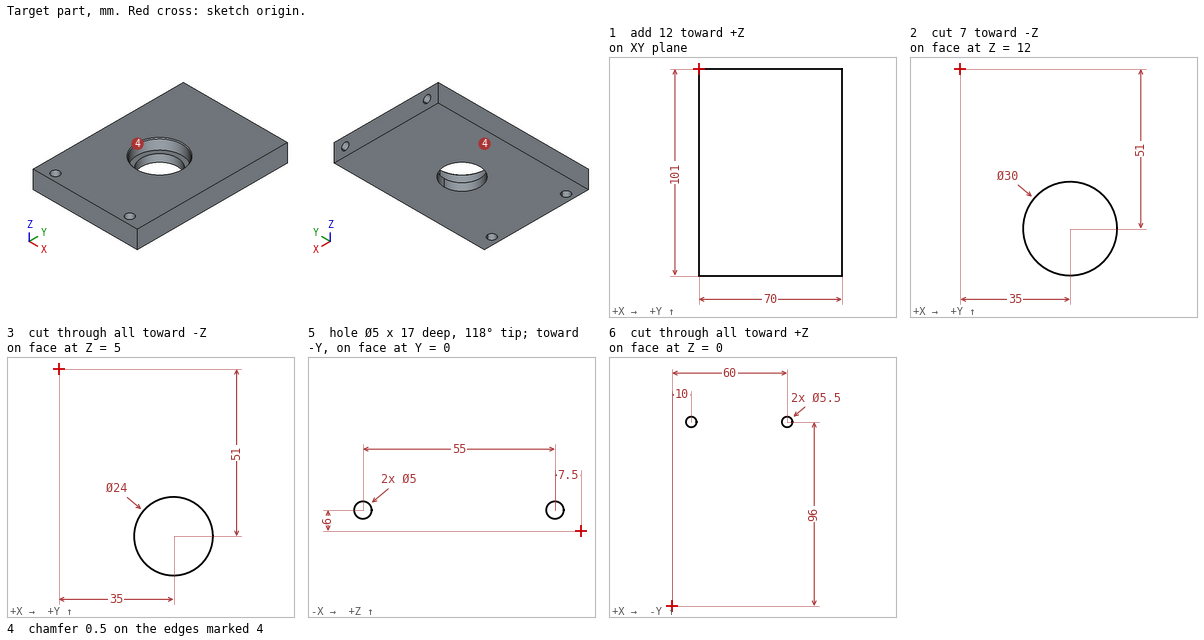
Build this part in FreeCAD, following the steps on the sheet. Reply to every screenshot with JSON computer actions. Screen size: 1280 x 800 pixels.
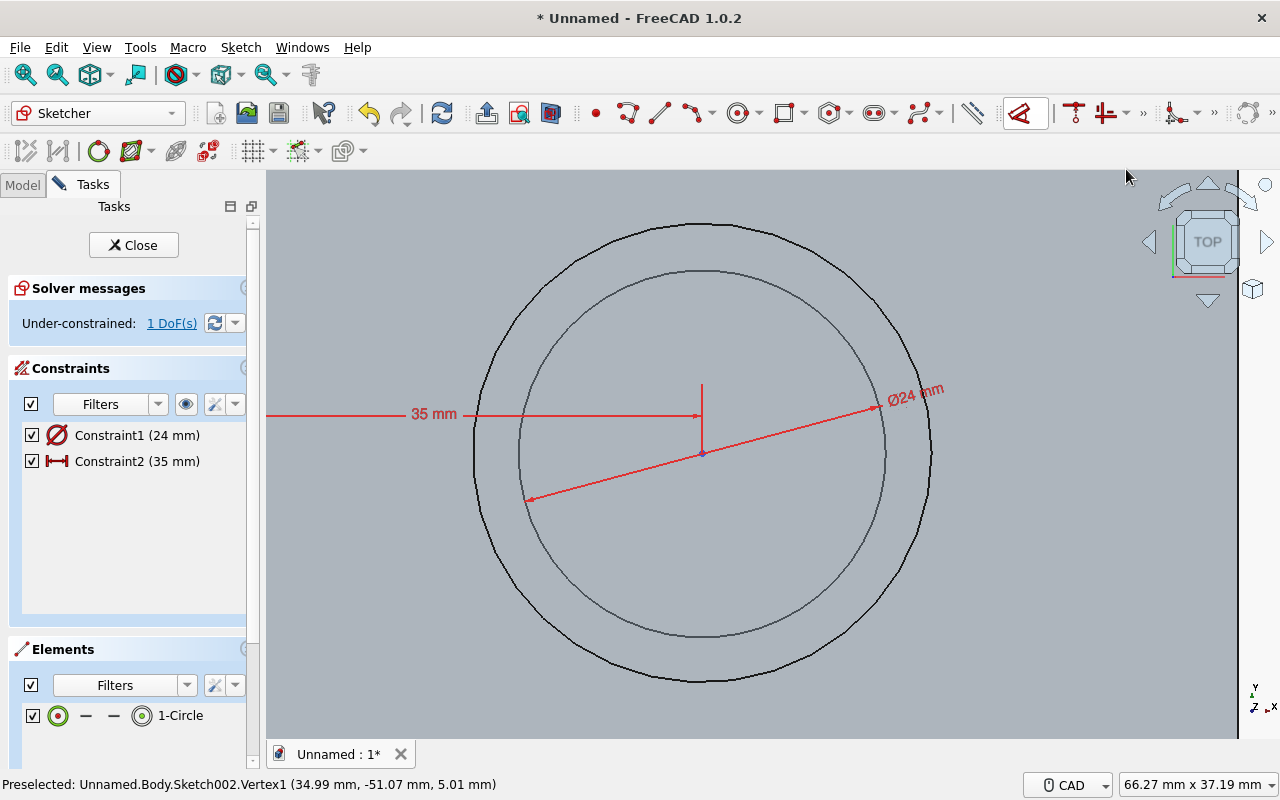
{"action": "left_click", "coordinate": [702, 454]}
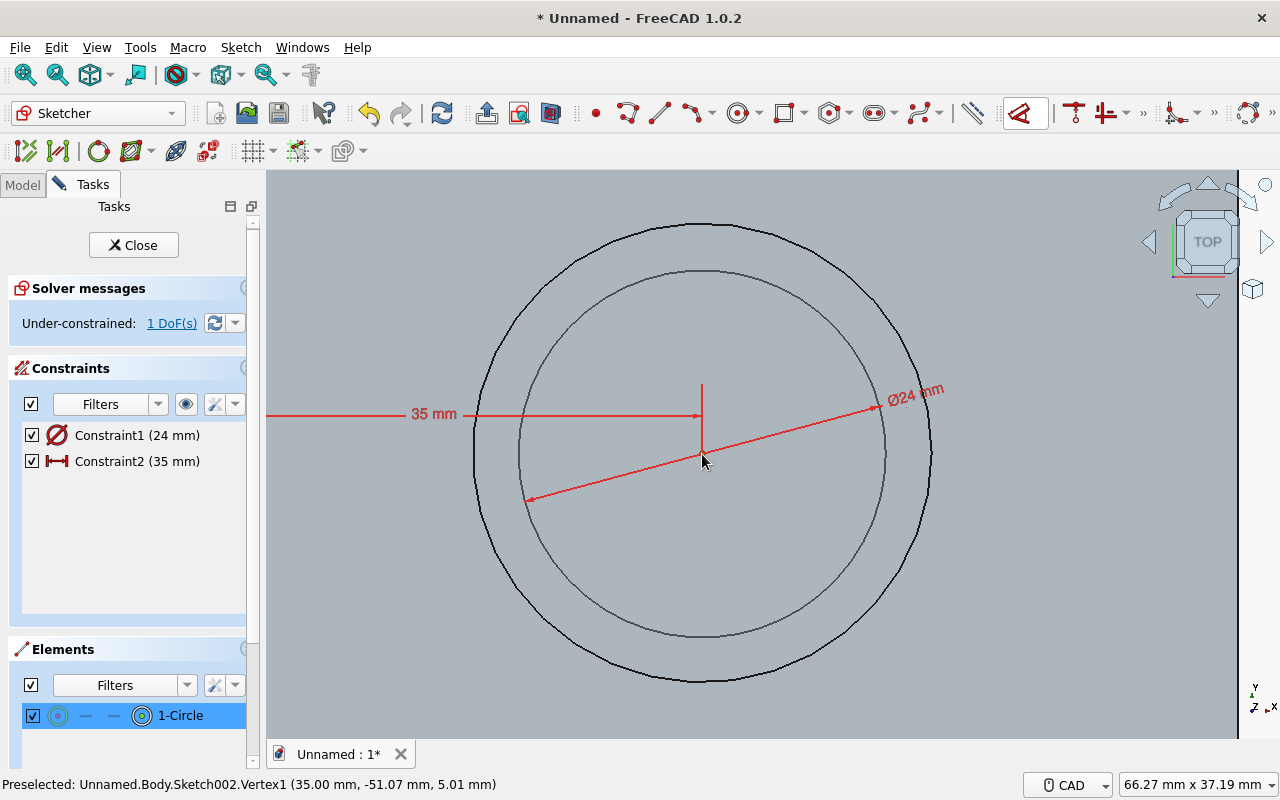
{"action": "left_click", "coordinate": [1042, 114]}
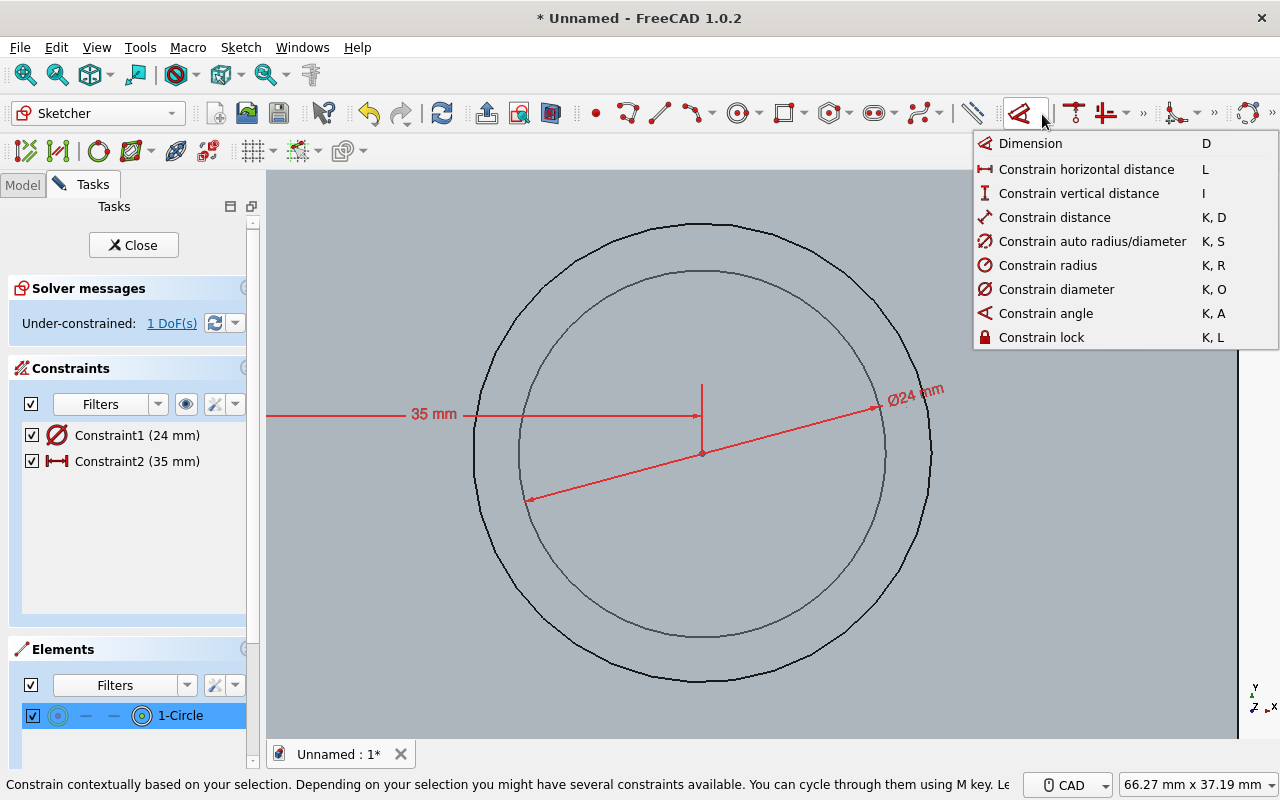
{"action": "left_click", "coordinate": [1126, 193]}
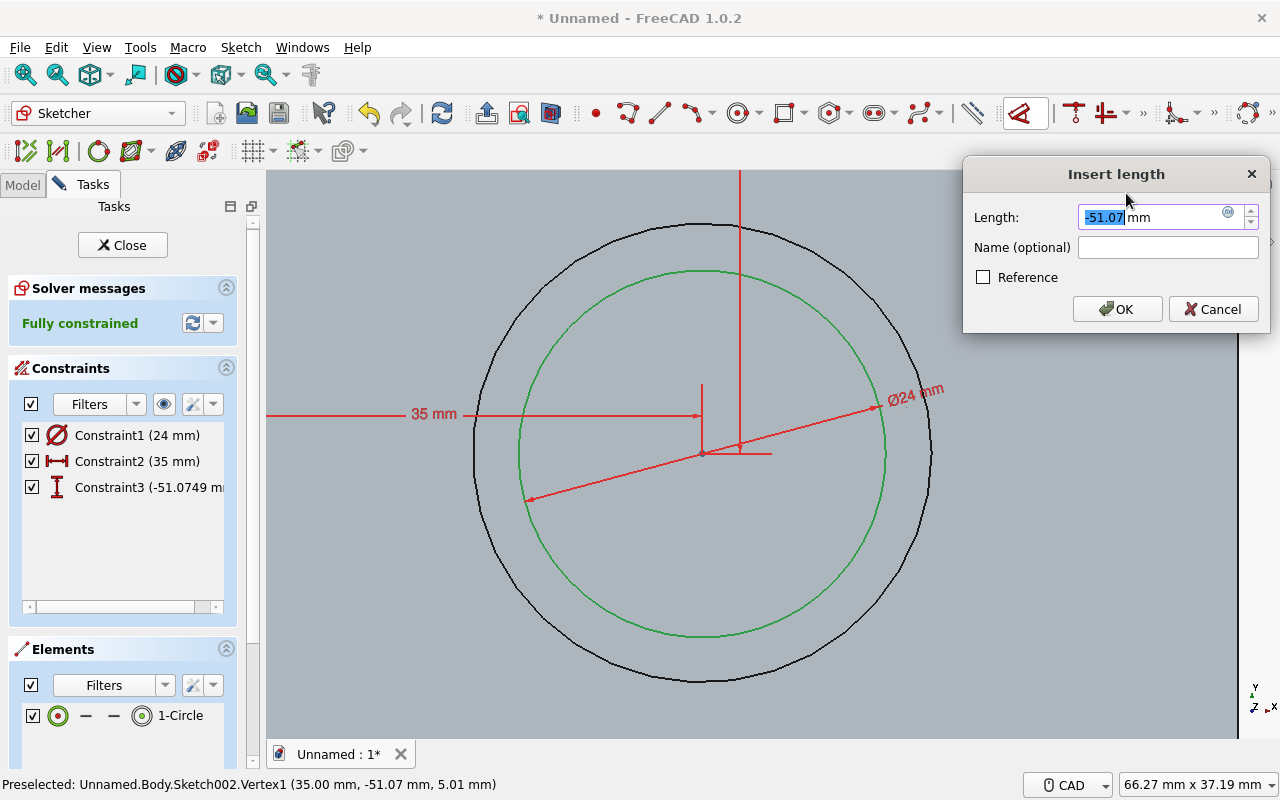
{"action": "type", "text": "-51"}
{"action": "key", "text": "Return"}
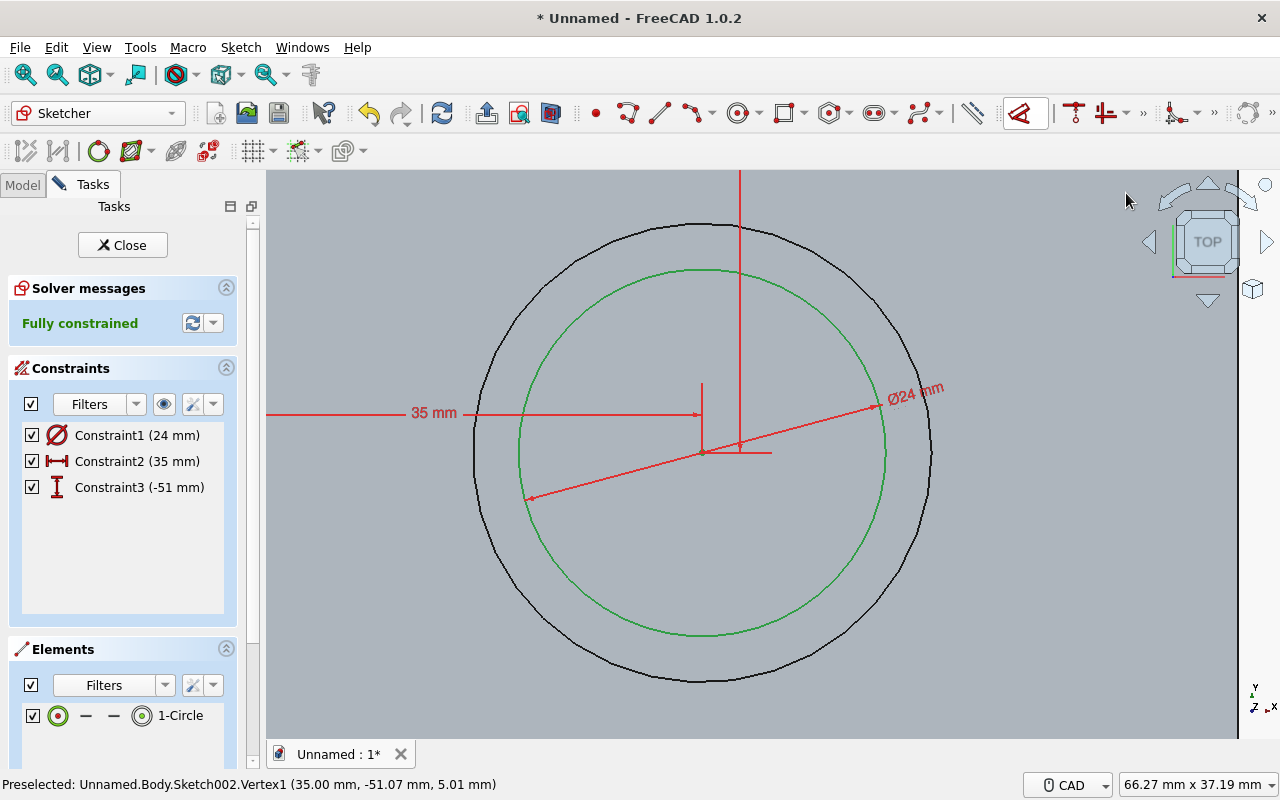
{"action": "left_click", "coordinate": [123, 245]}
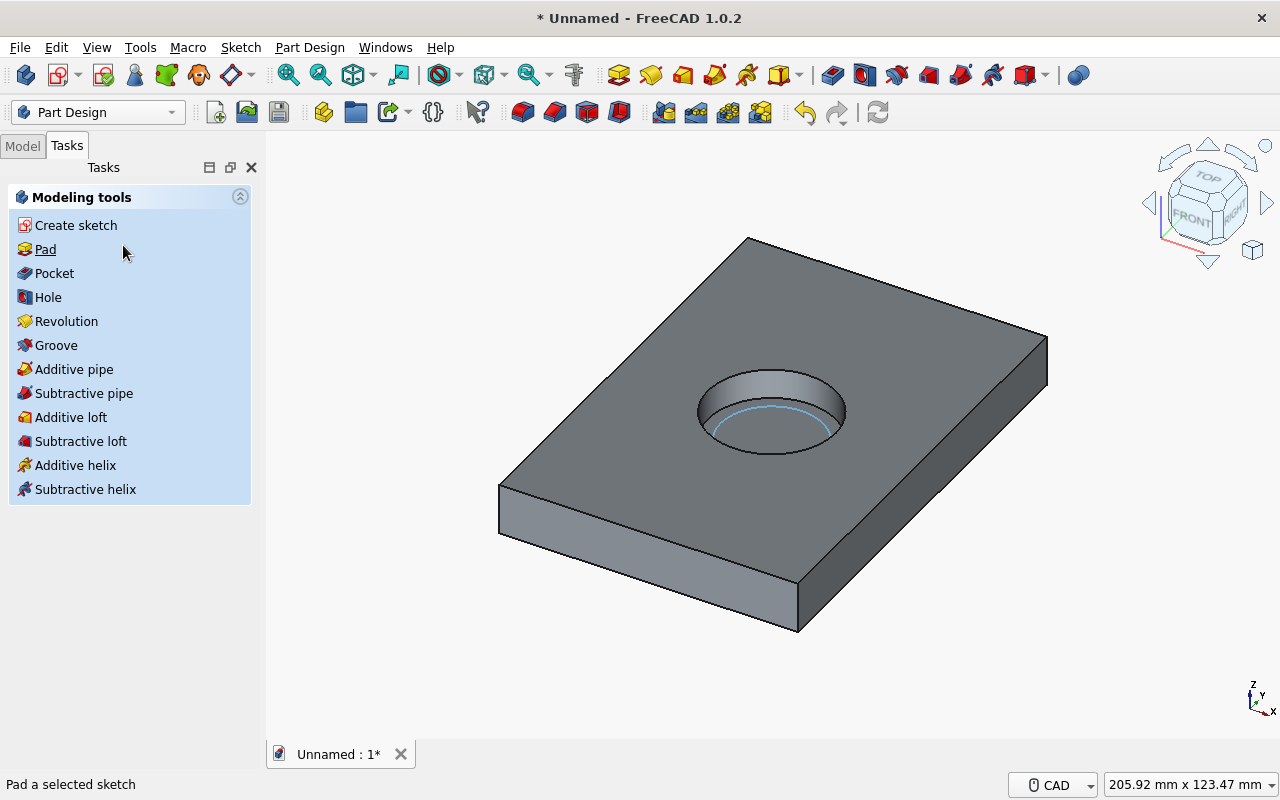
{"action": "left_click", "coordinate": [834, 76]}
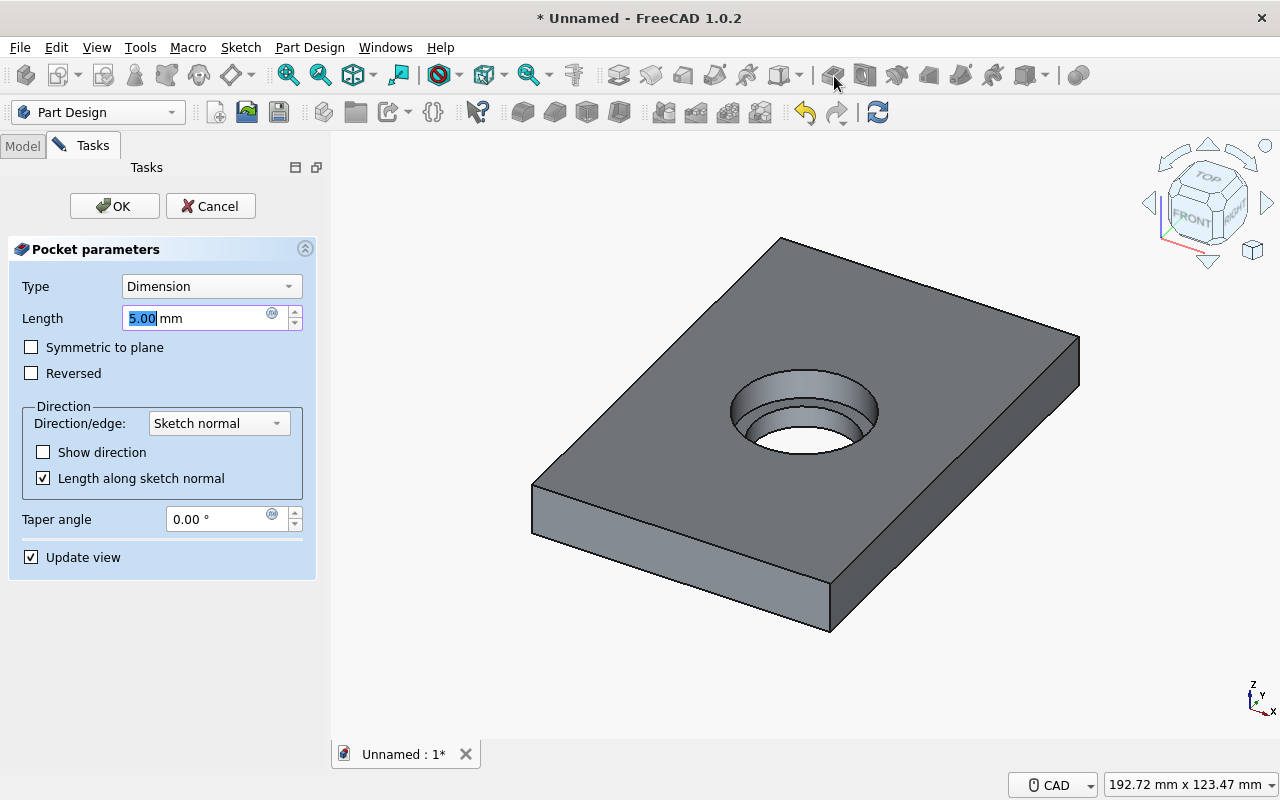
{"action": "left_click", "coordinate": [212, 286]}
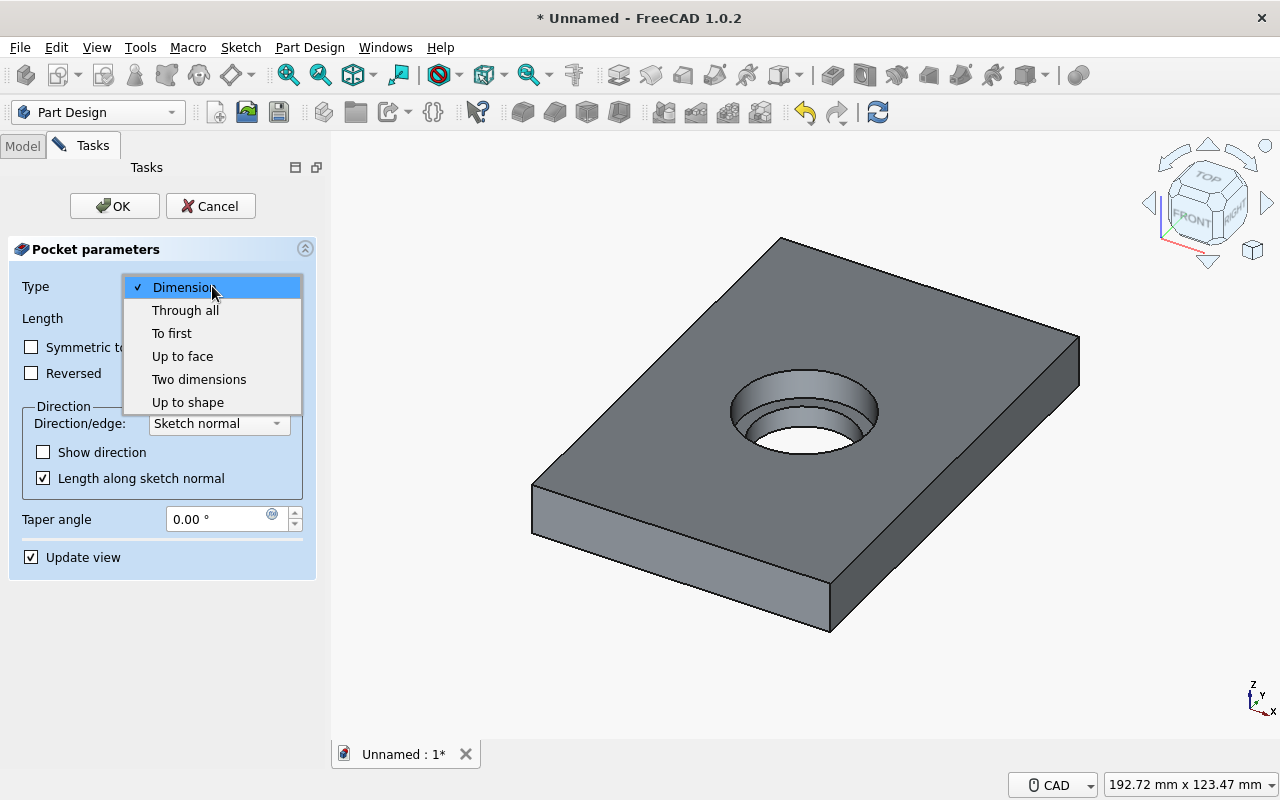
{"action": "left_click", "coordinate": [212, 310]}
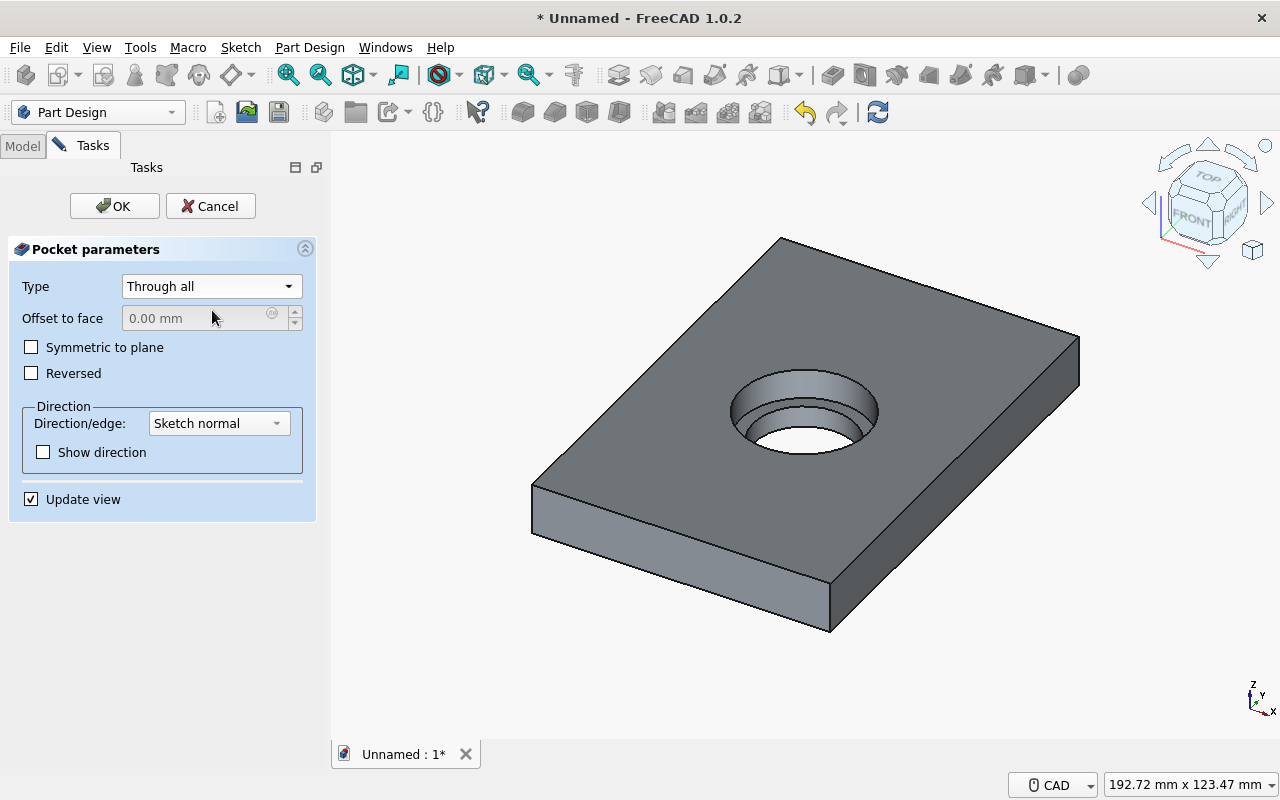
{"action": "left_click", "coordinate": [115, 206]}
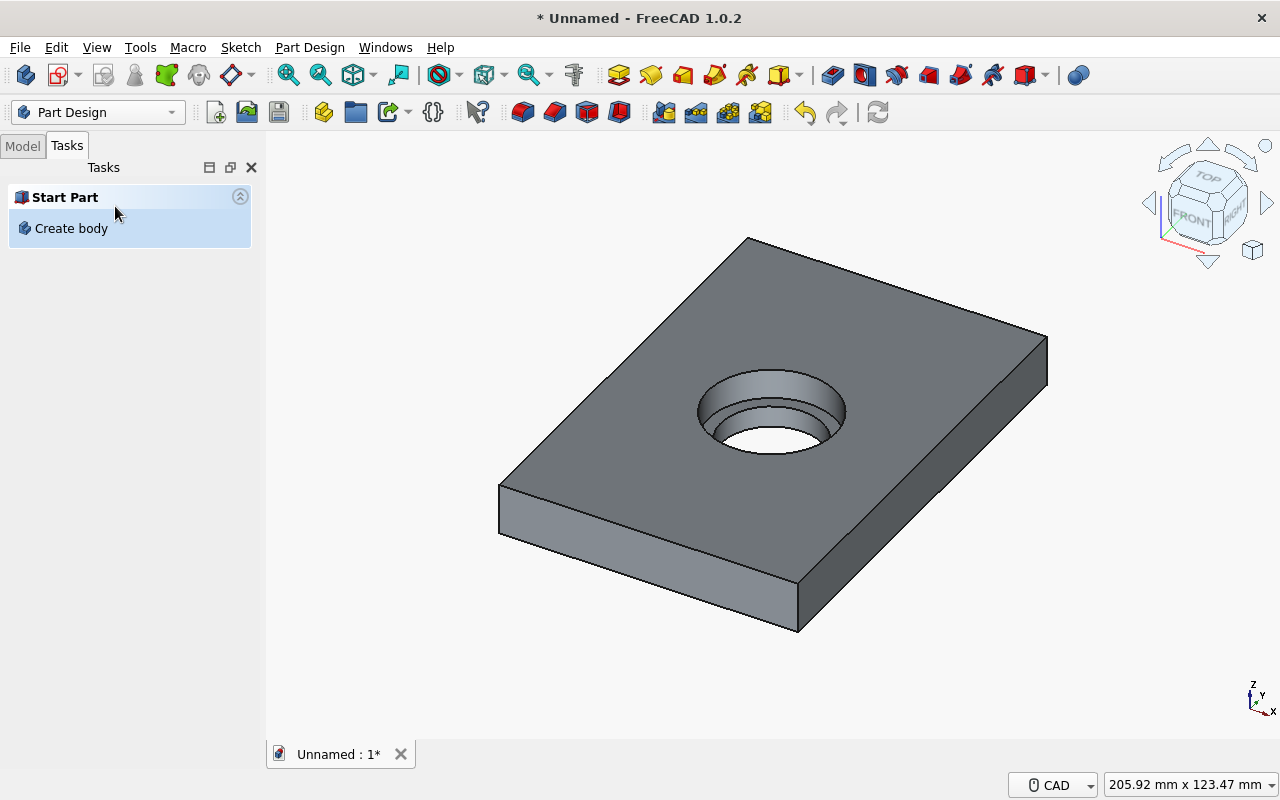
{"action": "left_click", "coordinate": [708, 390]}